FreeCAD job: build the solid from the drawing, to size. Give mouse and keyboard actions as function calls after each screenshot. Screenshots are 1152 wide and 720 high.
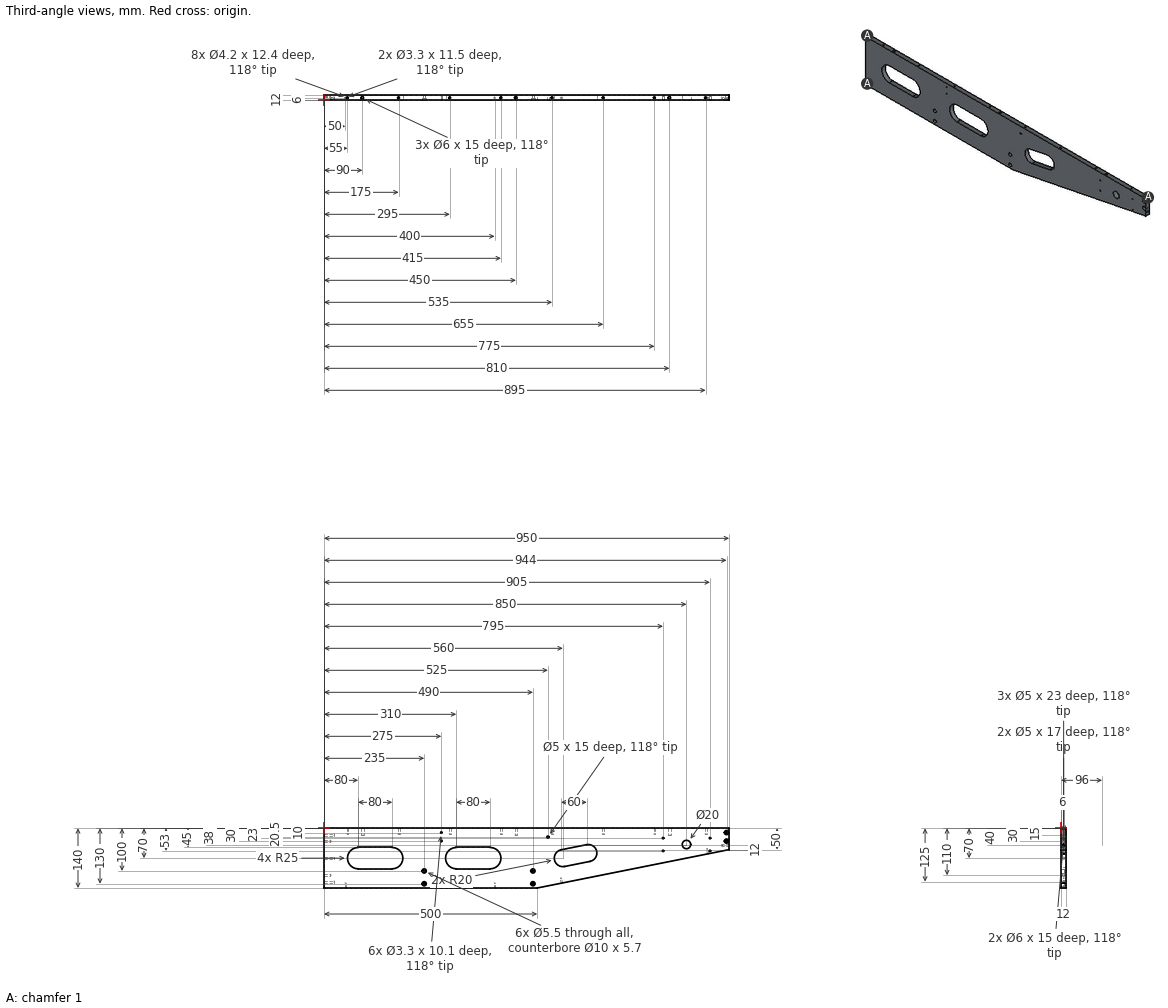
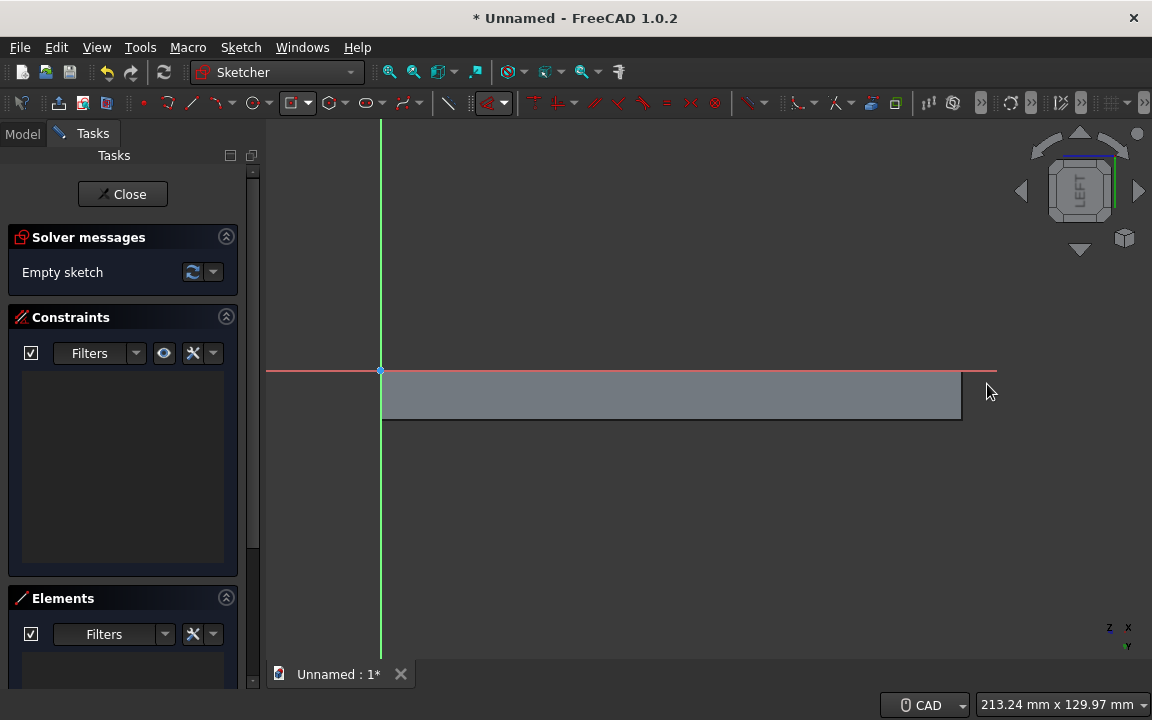
click(254, 104)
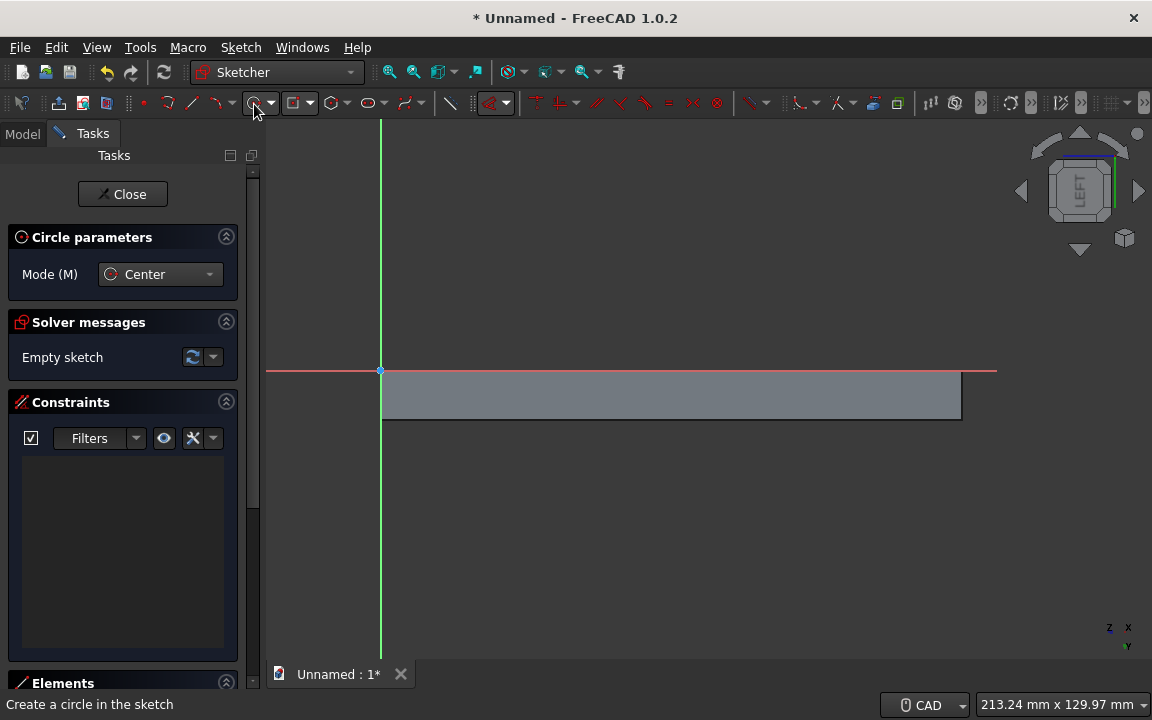
scroll(443, 395, up, 4)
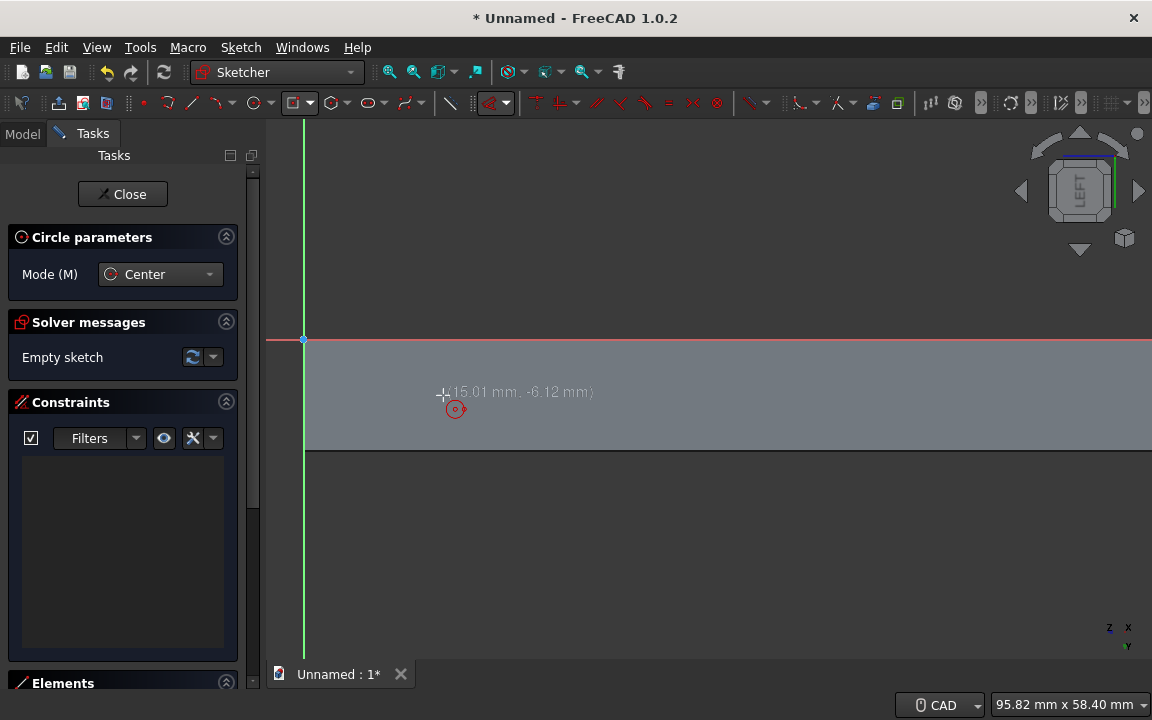
click(443, 395)
move(459, 379)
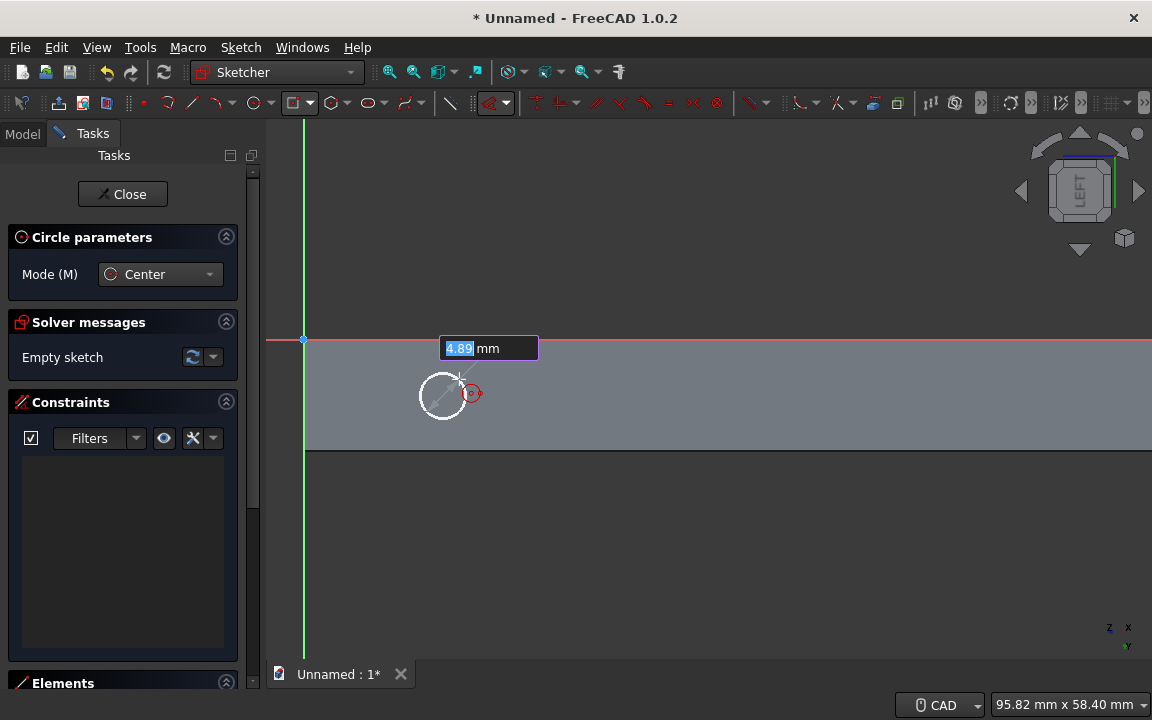
text(5)
key(Return)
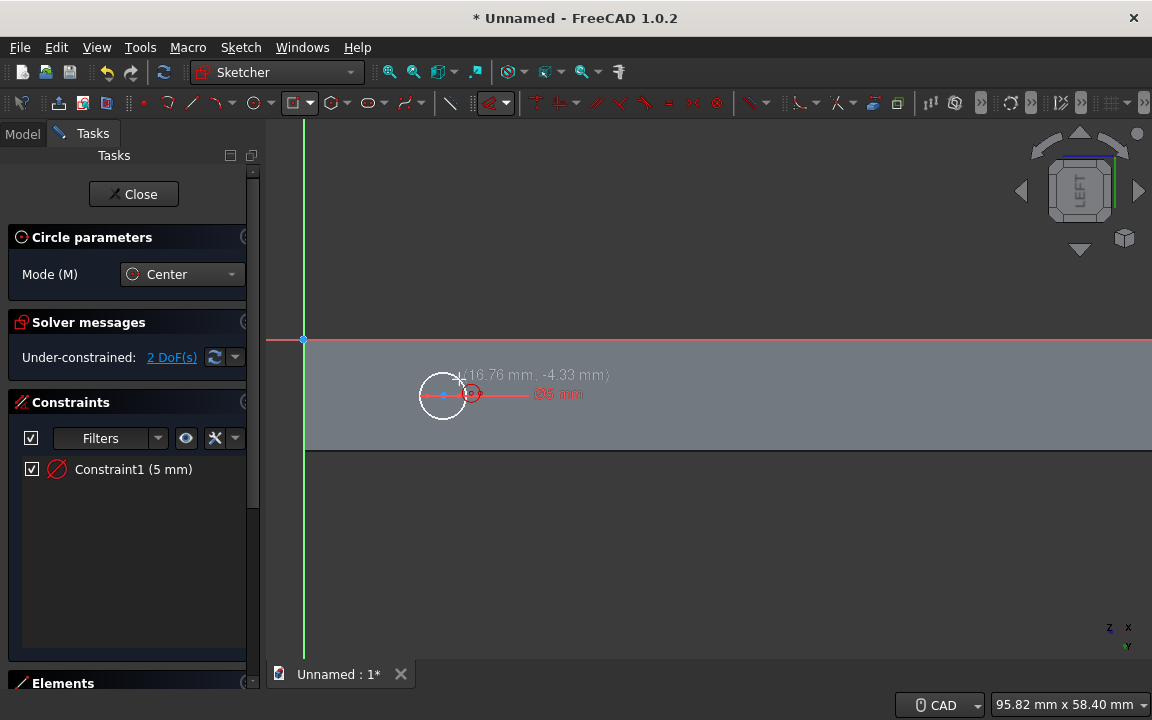
click(951, 395)
move(968, 379)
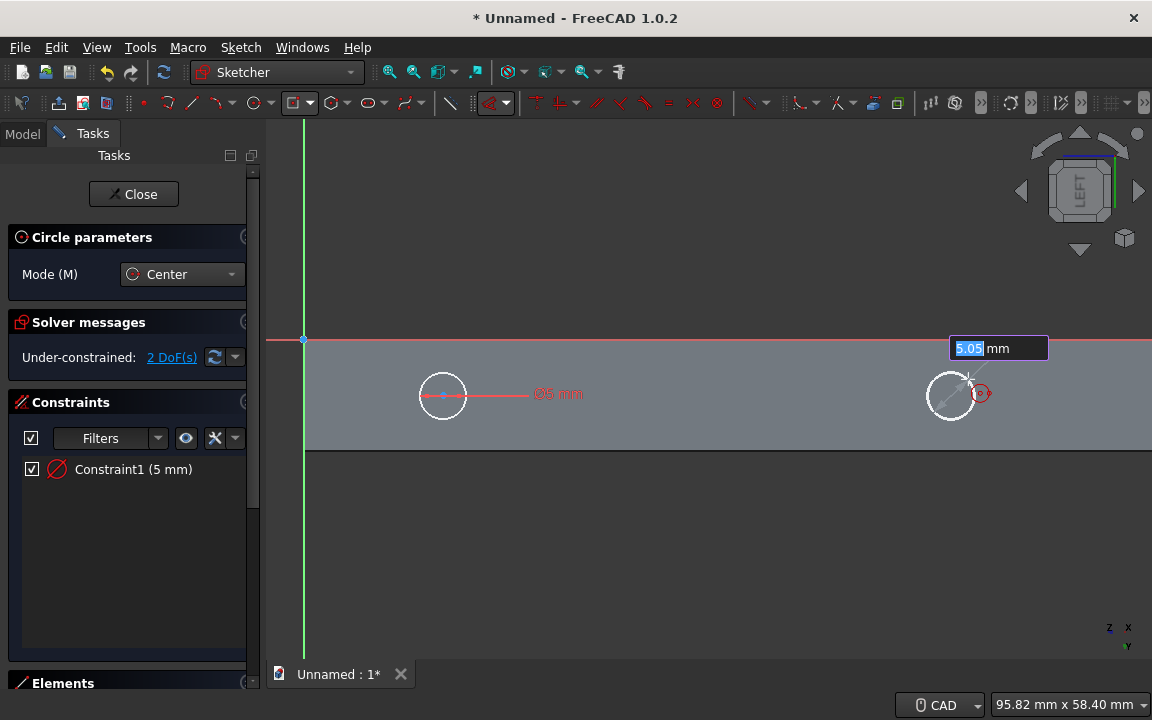
text(5)
key(Return)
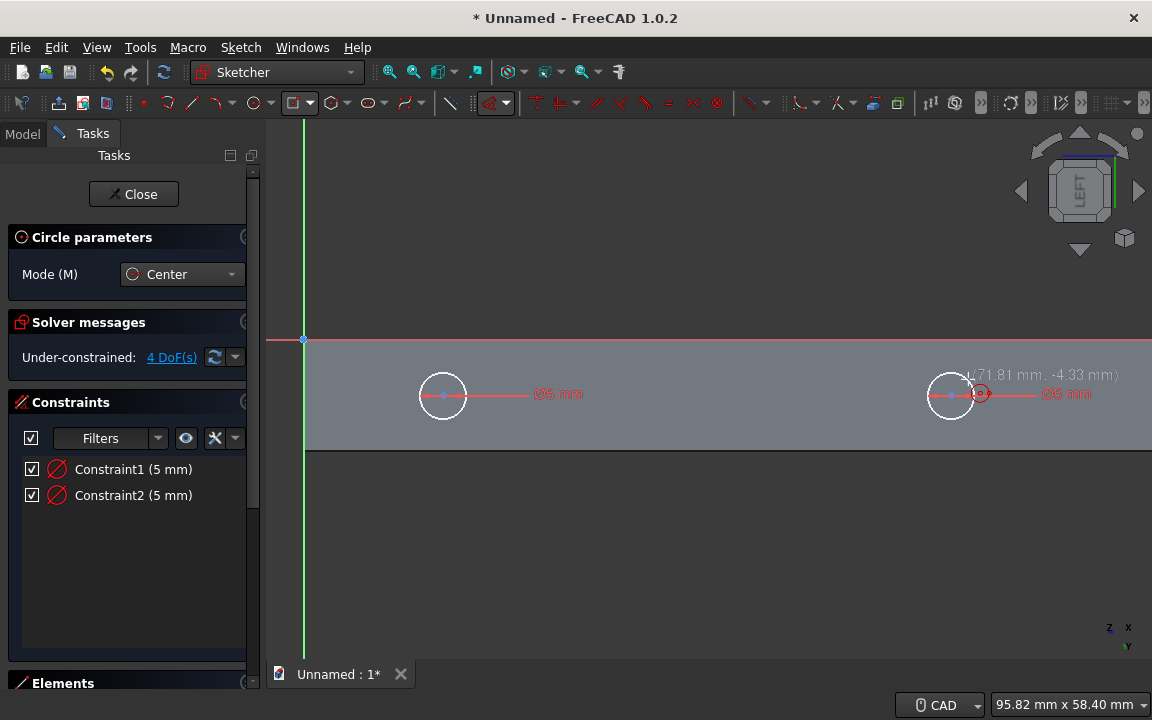
scroll(434, 397, down, 4)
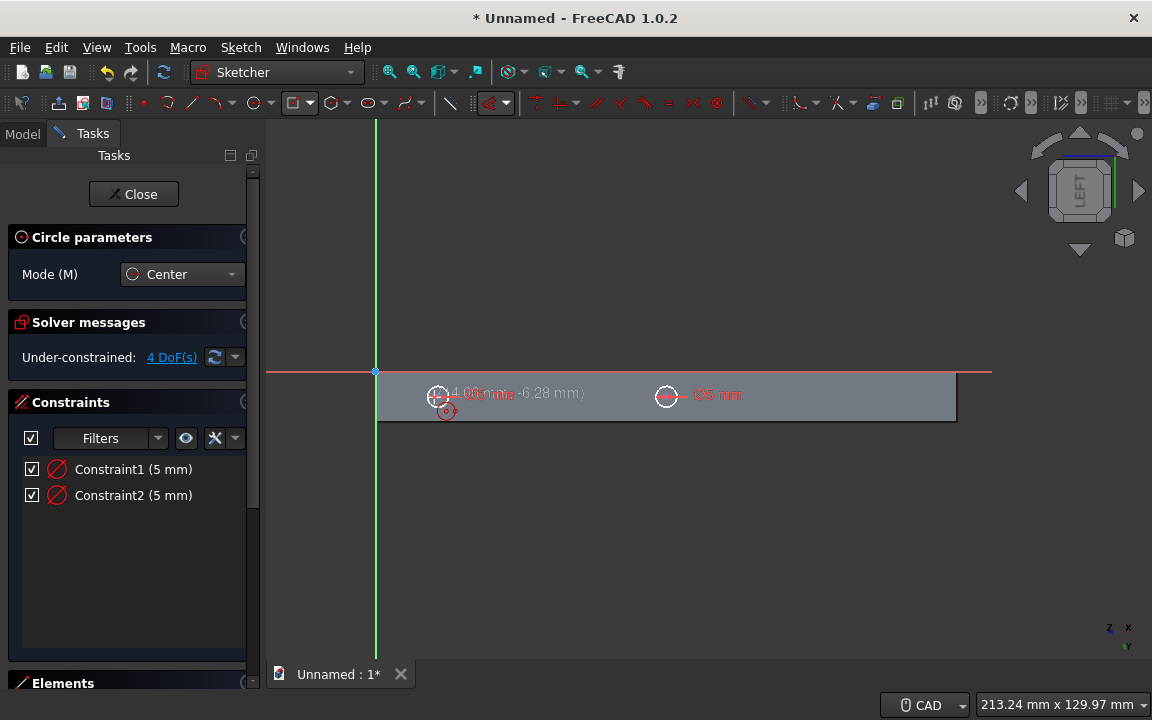
scroll(895, 397, up, 4)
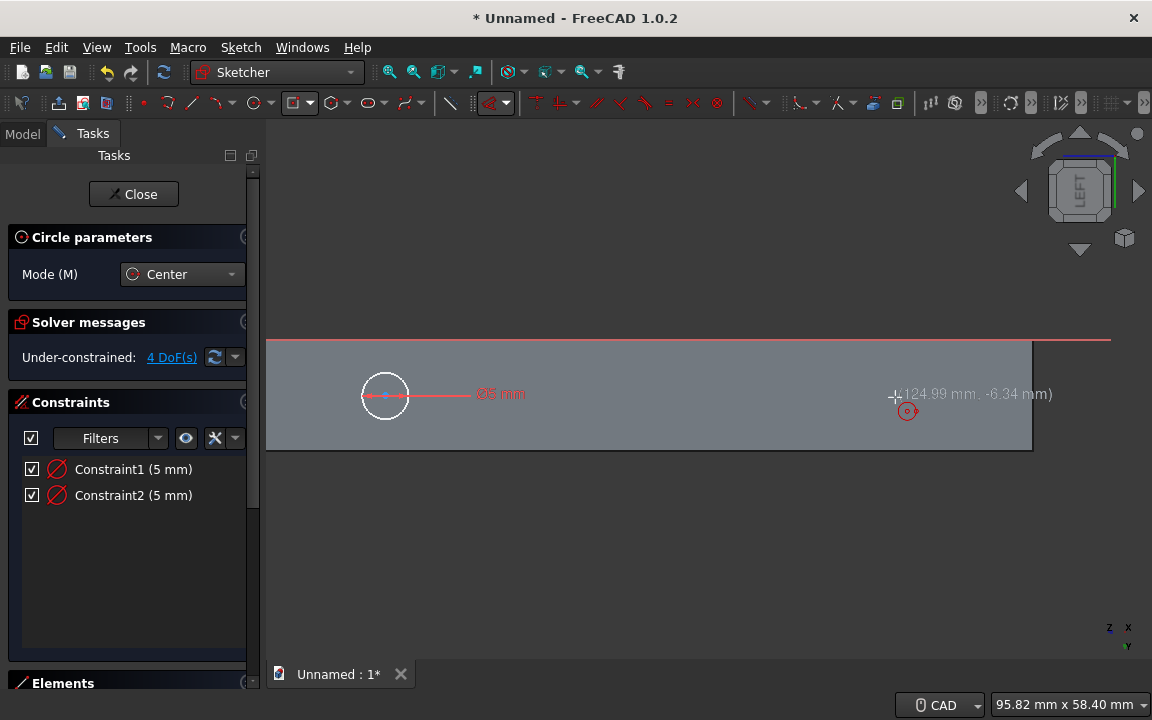
click(894, 395)
move(911, 379)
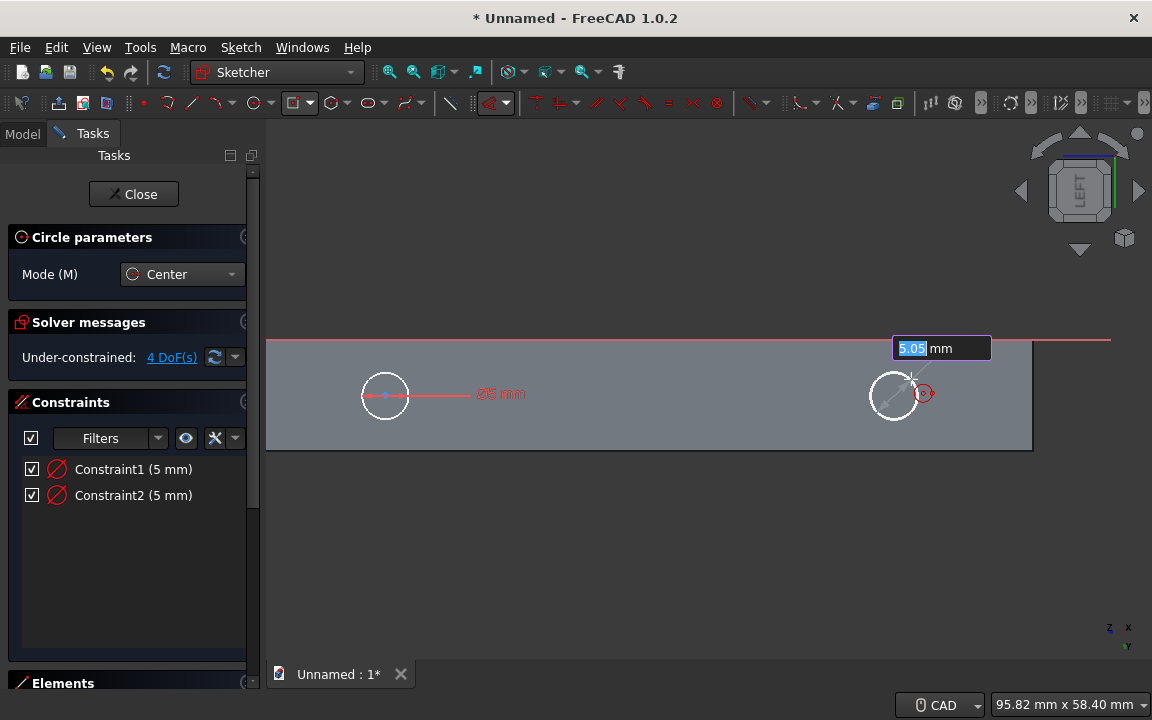
text(5)
key(Return)
key(Escape)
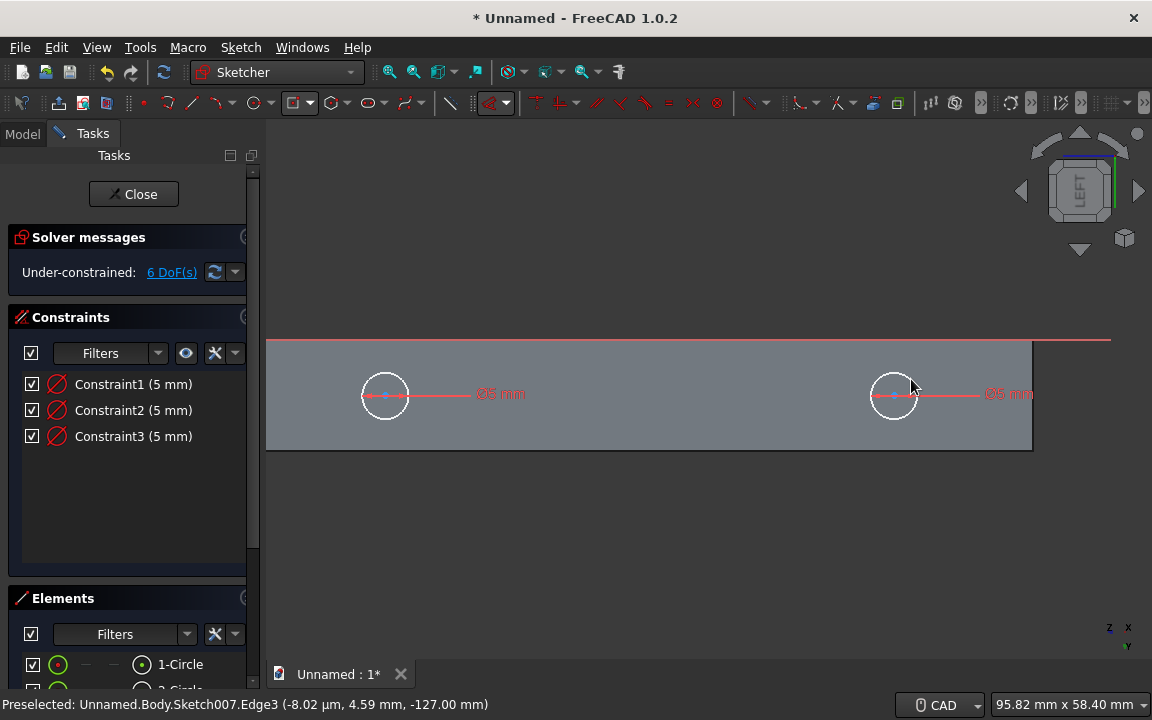
scroll(896, 397, down, 4)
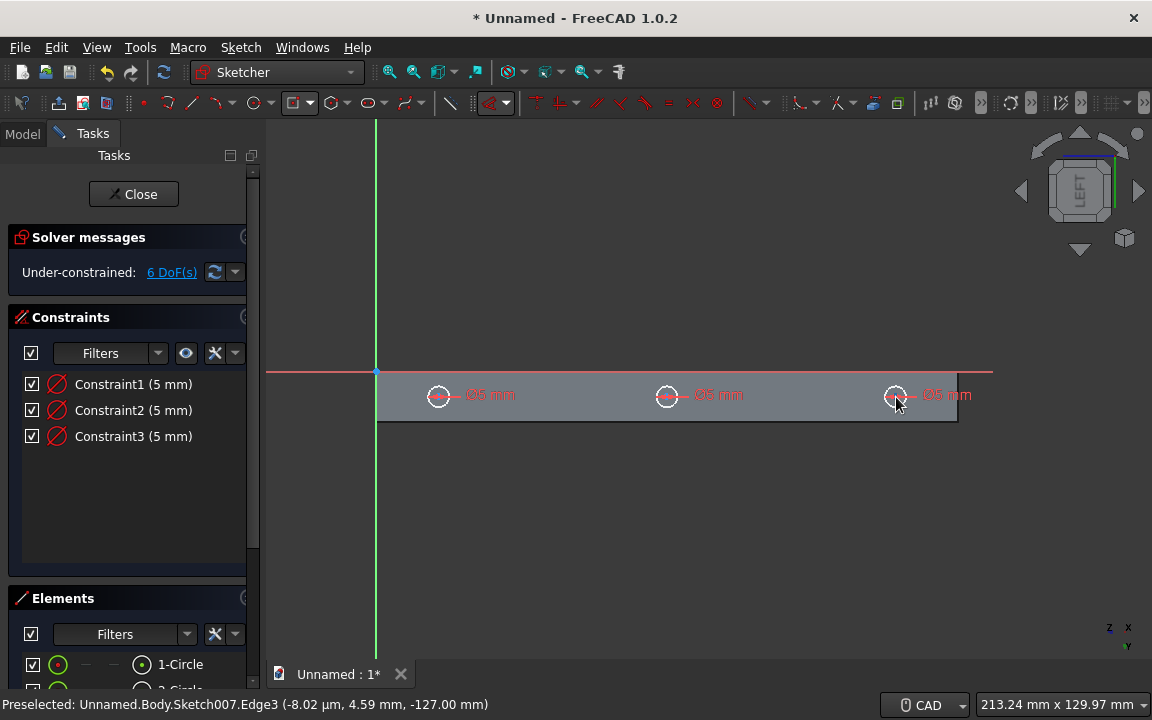
click(439, 397)